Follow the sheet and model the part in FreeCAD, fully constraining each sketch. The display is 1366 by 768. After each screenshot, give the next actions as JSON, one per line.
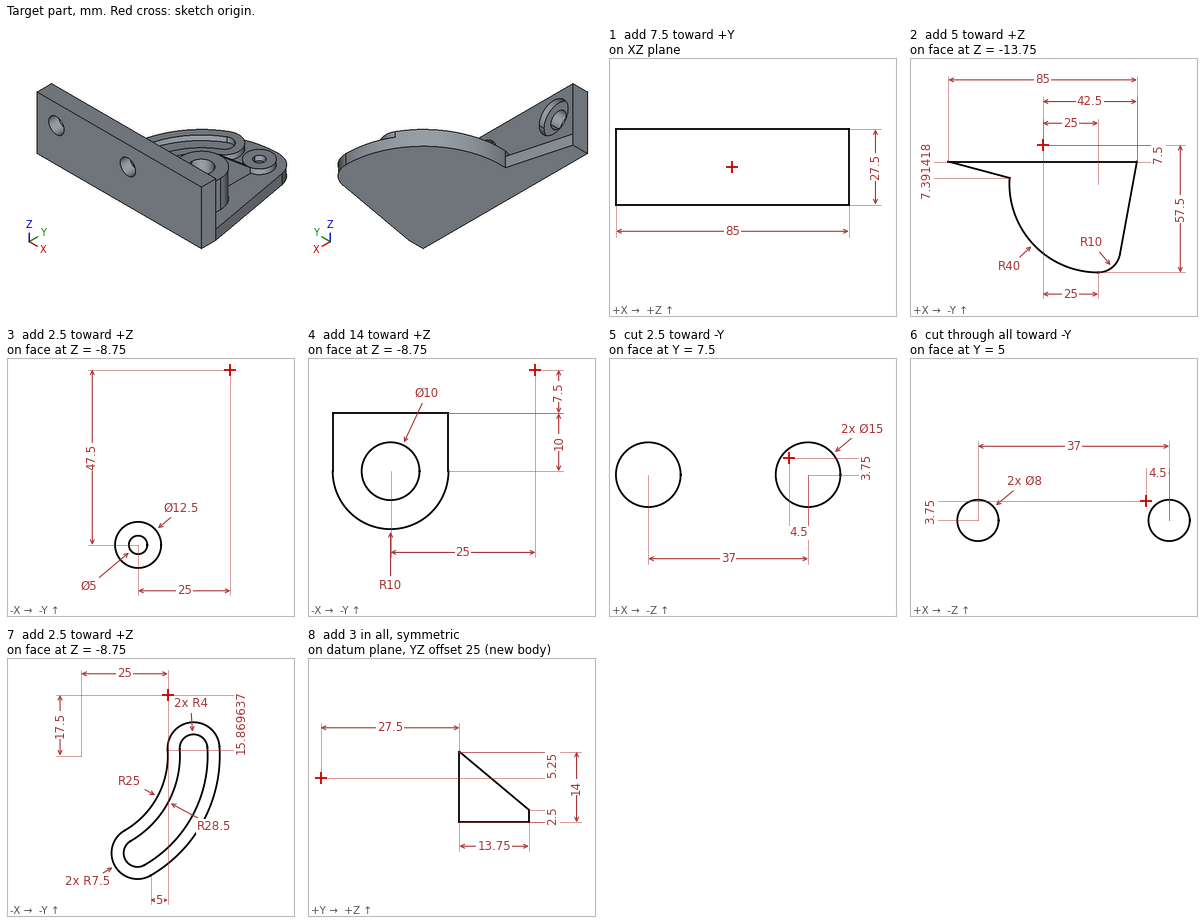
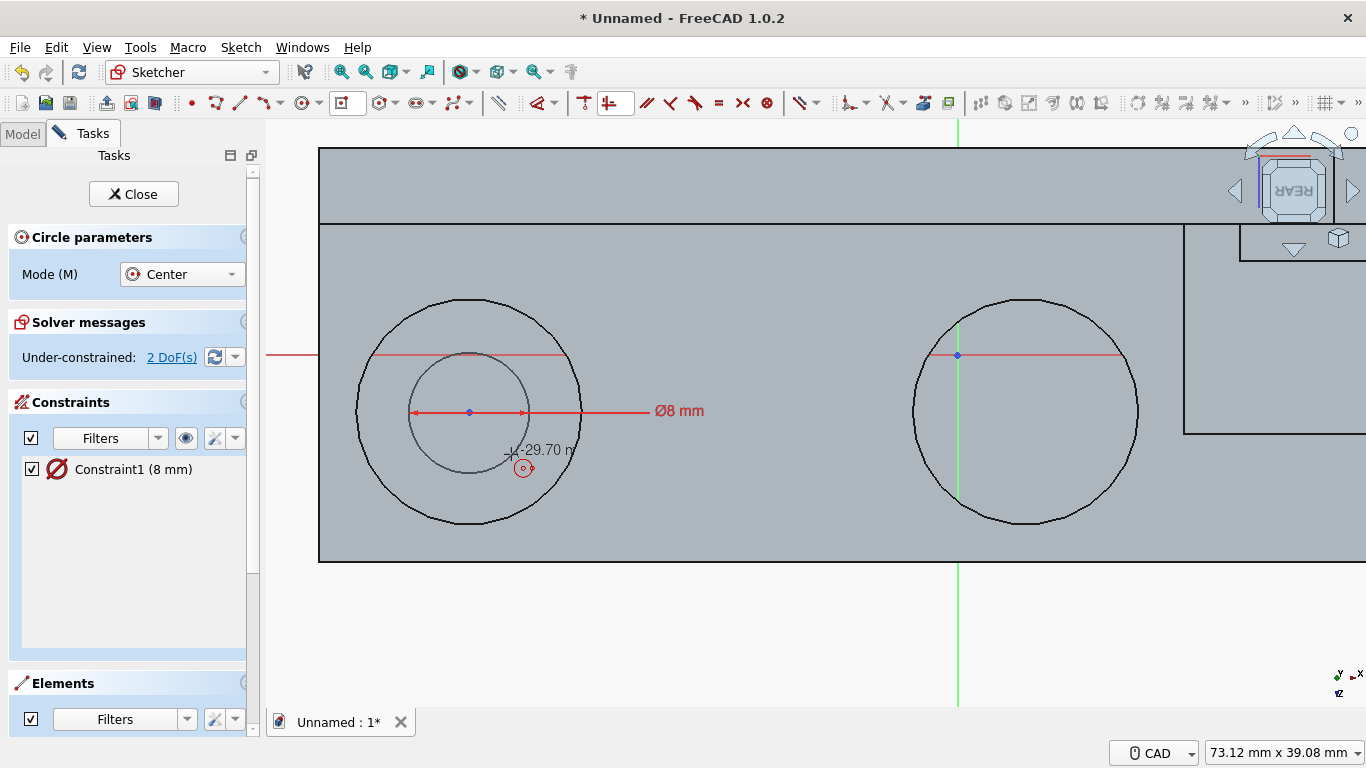
{"action": "left_click", "coordinate": [1026, 412]}
{"action": "mouse_move", "coordinate": [1068, 454]}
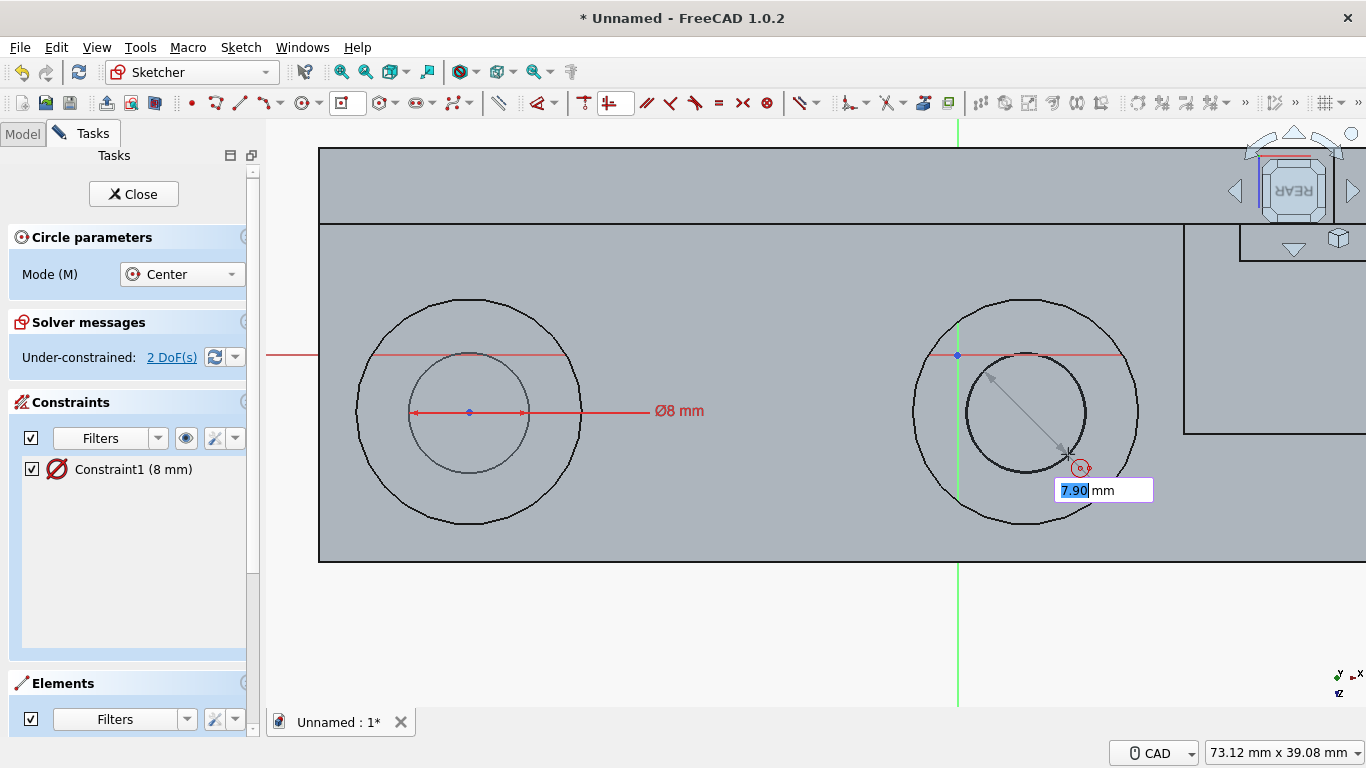
{"action": "type", "text": "8"}
{"action": "key", "text": "Return"}
{"action": "key", "text": "Escape"}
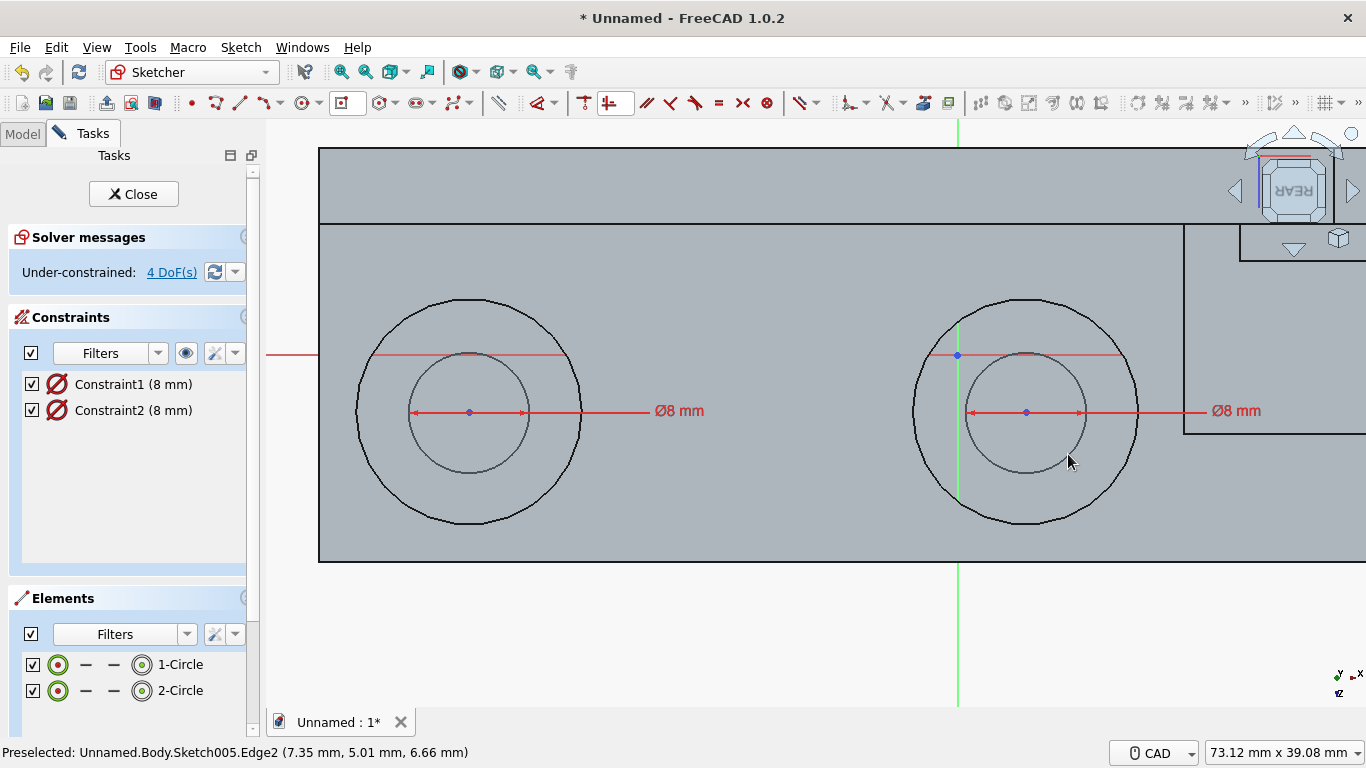
{"action": "left_click", "coordinate": [469, 413]}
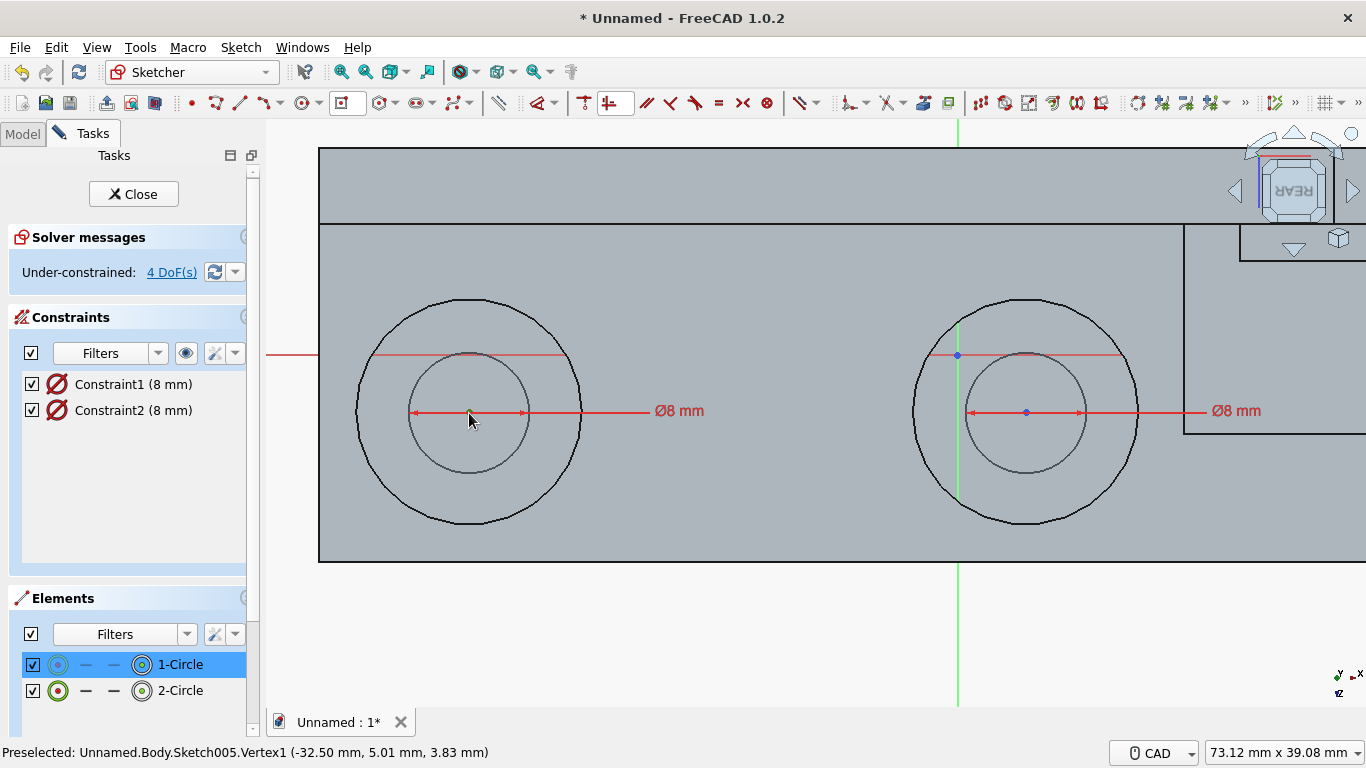
{"action": "left_click", "coordinate": [1026, 413]}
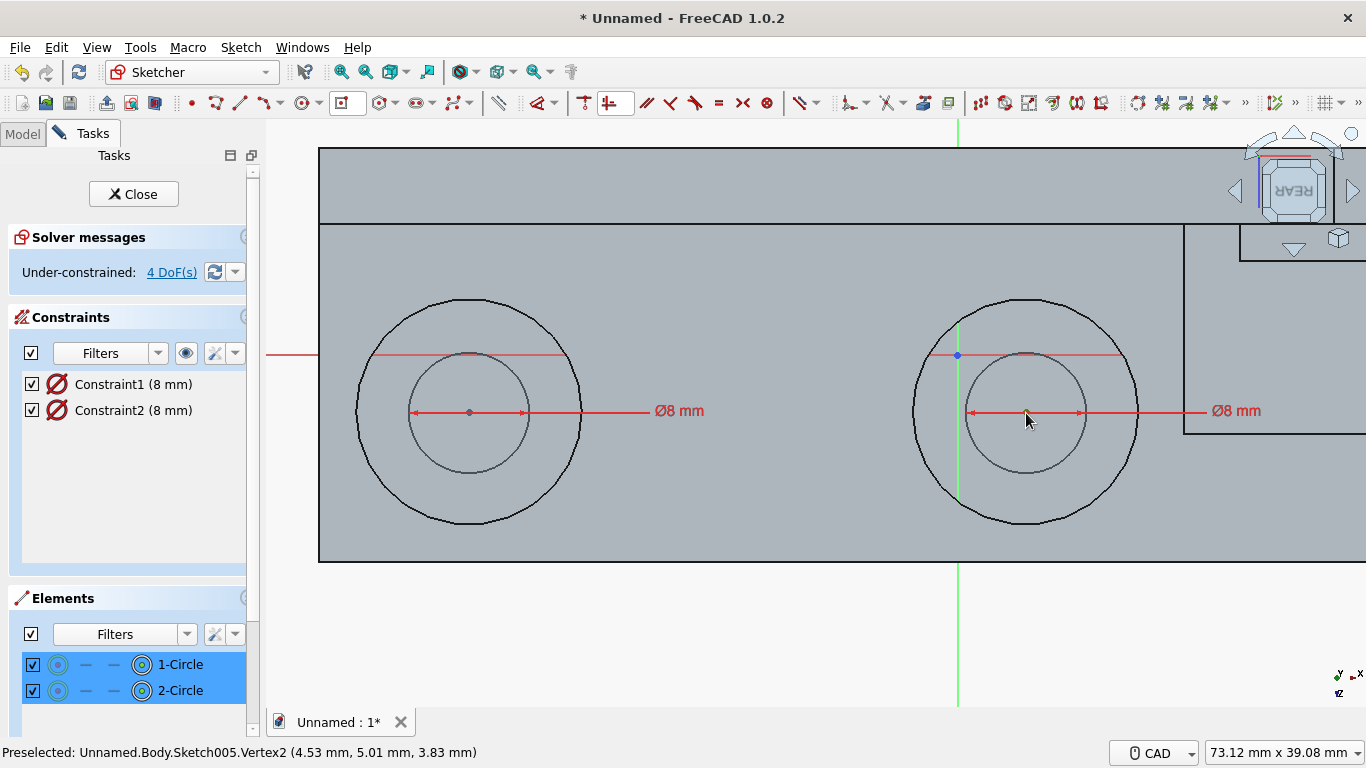
{"action": "key", "text": "h"}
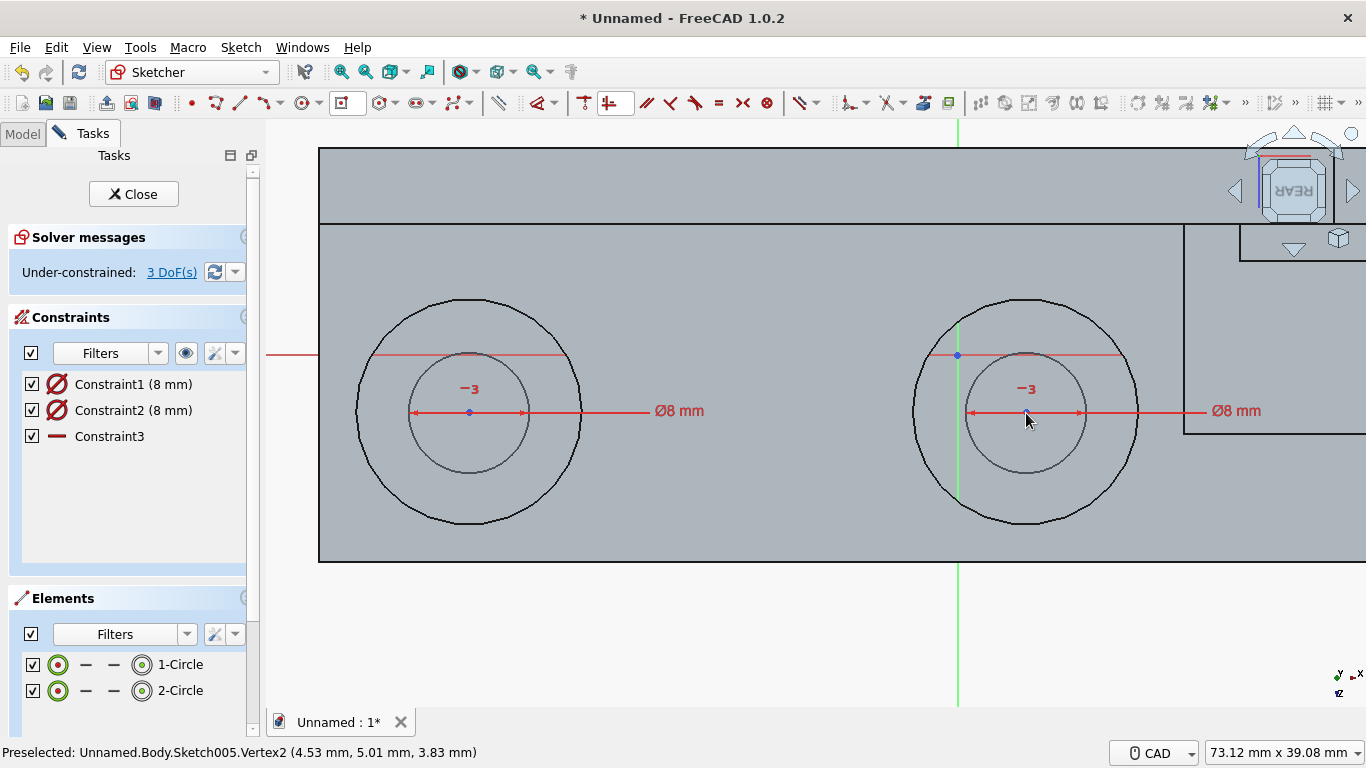
{"action": "left_click", "coordinate": [538, 104]}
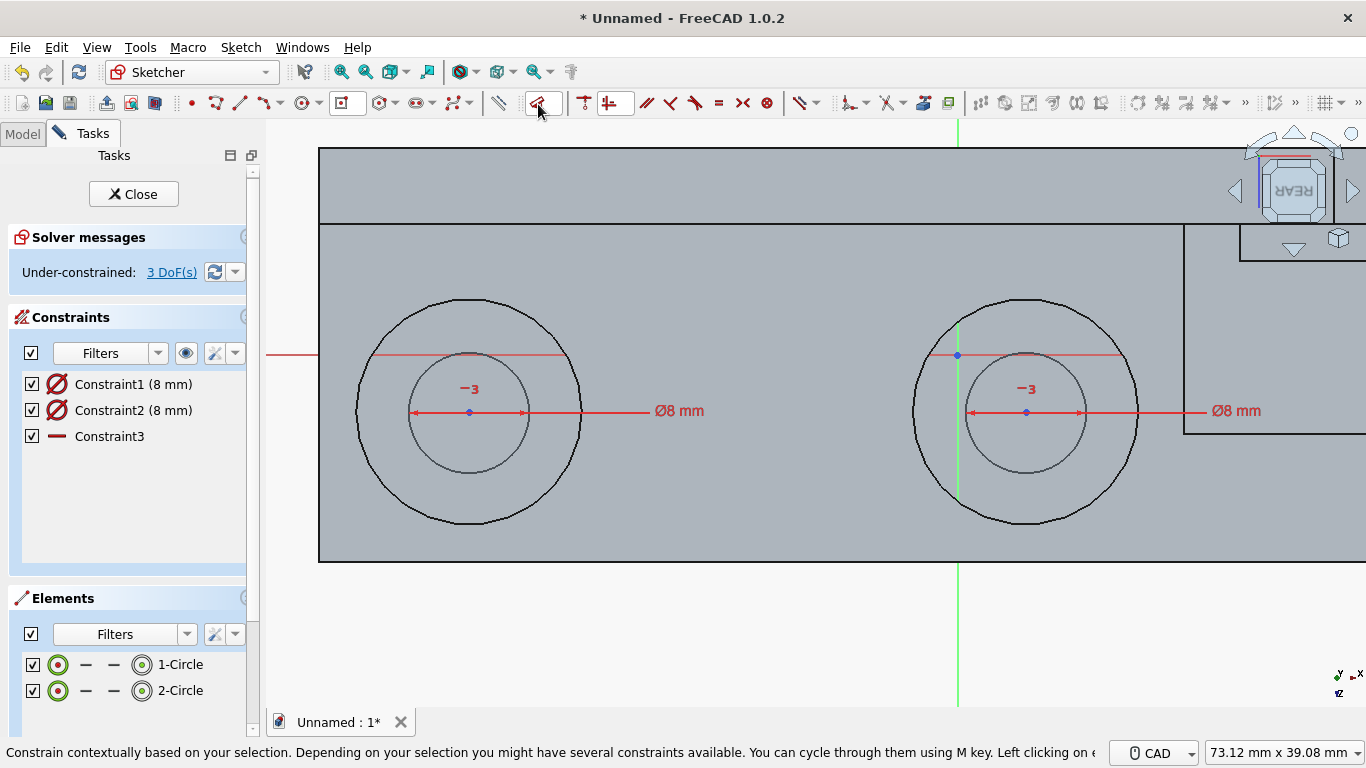
{"action": "left_click", "coordinate": [1026, 413]}
{"action": "left_click", "coordinate": [992, 321]}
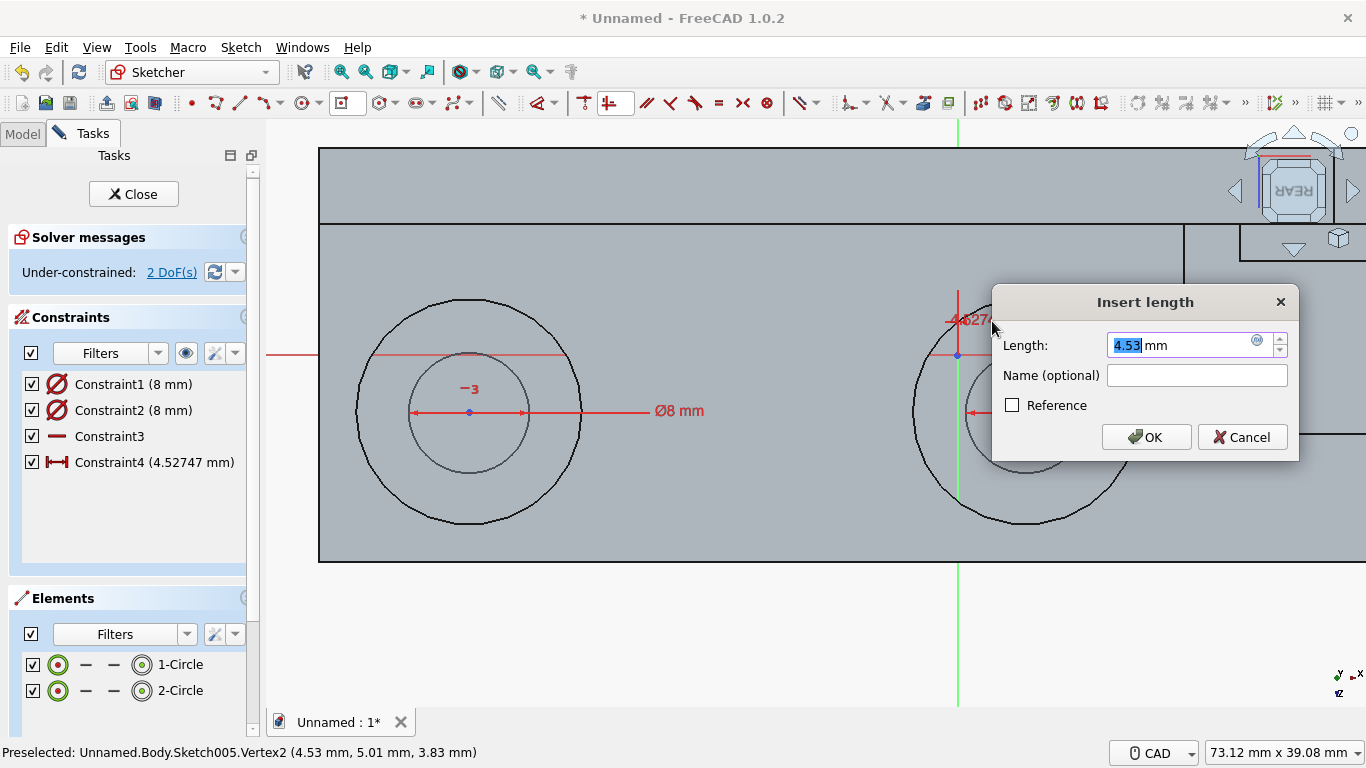
{"action": "type", "text": "4.5"}
{"action": "key", "text": "Return"}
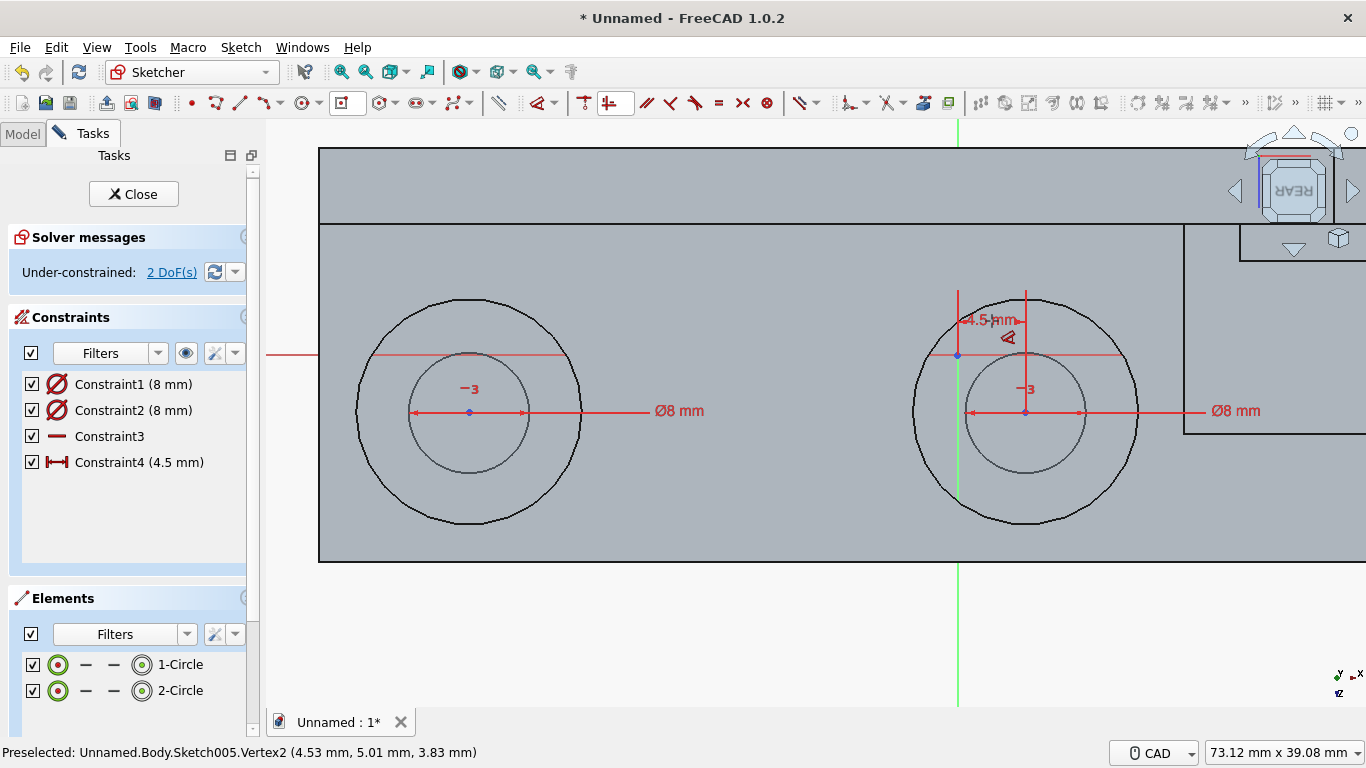
{"action": "left_click", "coordinate": [469, 413]}